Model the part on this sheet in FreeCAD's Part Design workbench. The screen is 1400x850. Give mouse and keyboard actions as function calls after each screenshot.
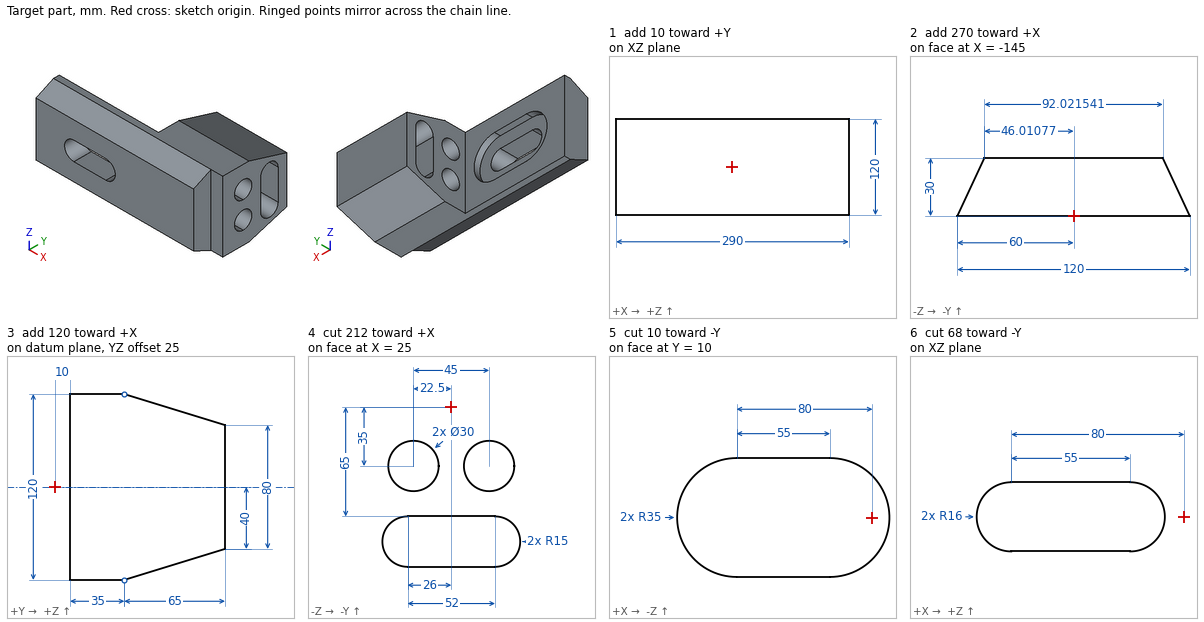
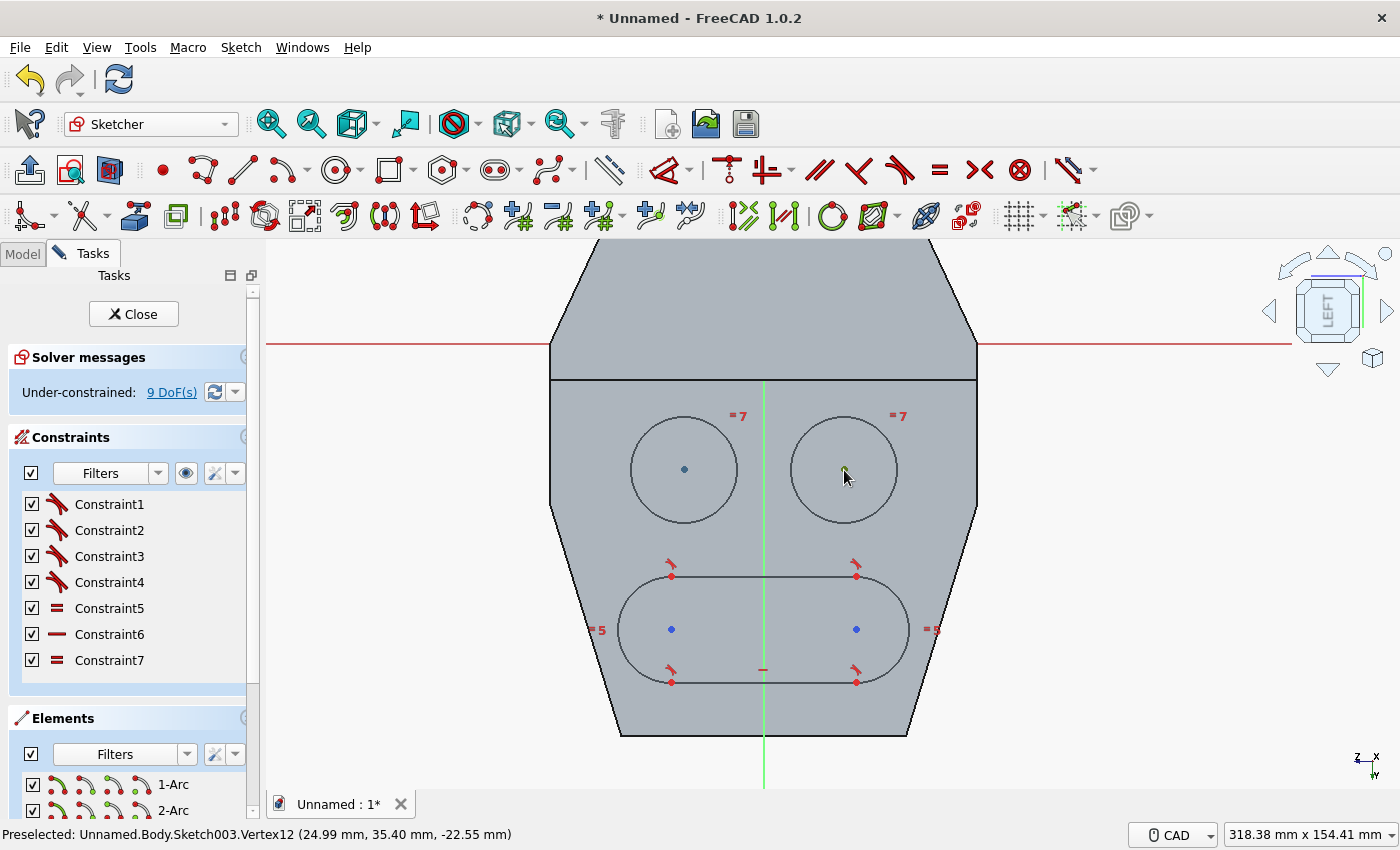
key(h)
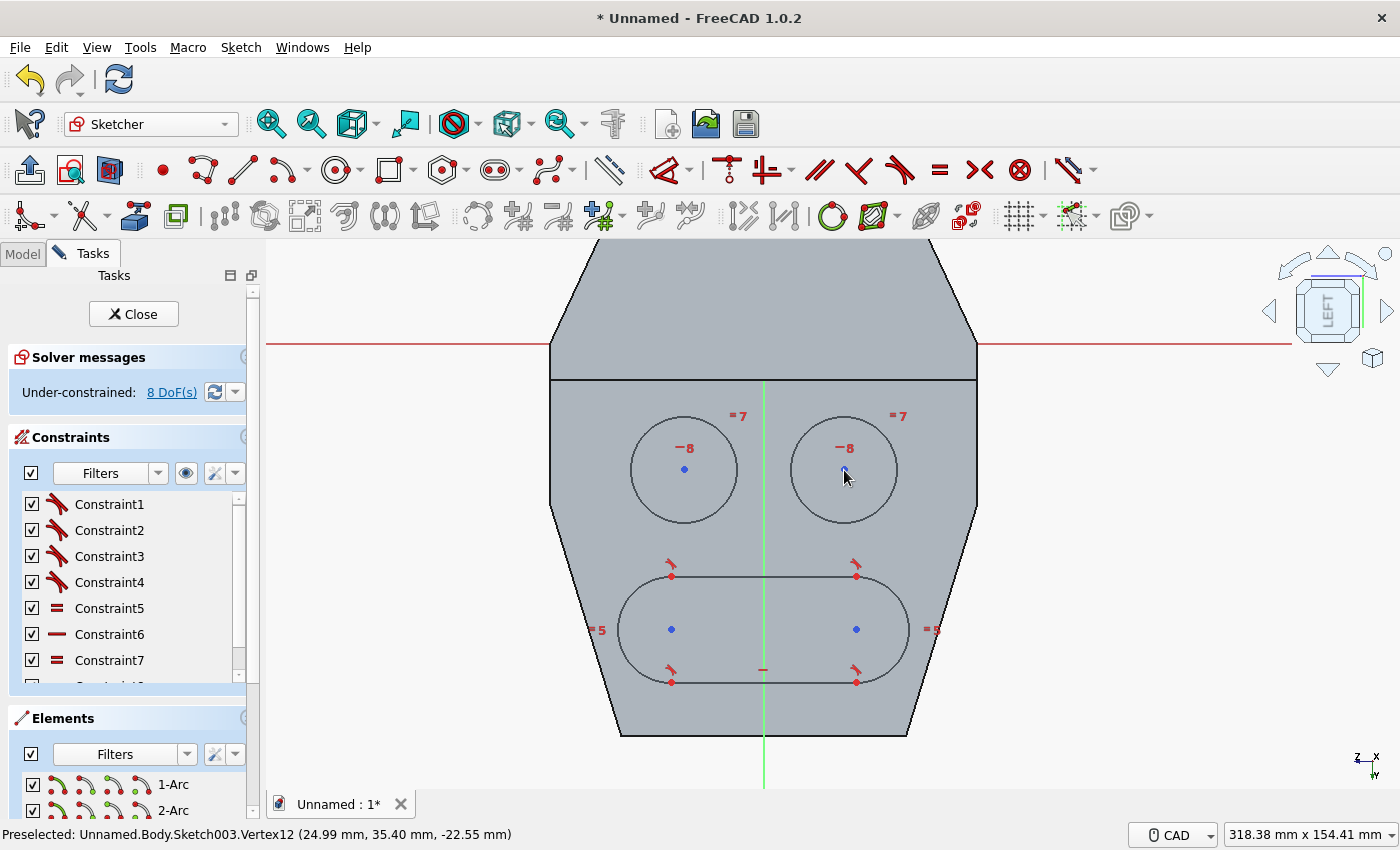
key(d)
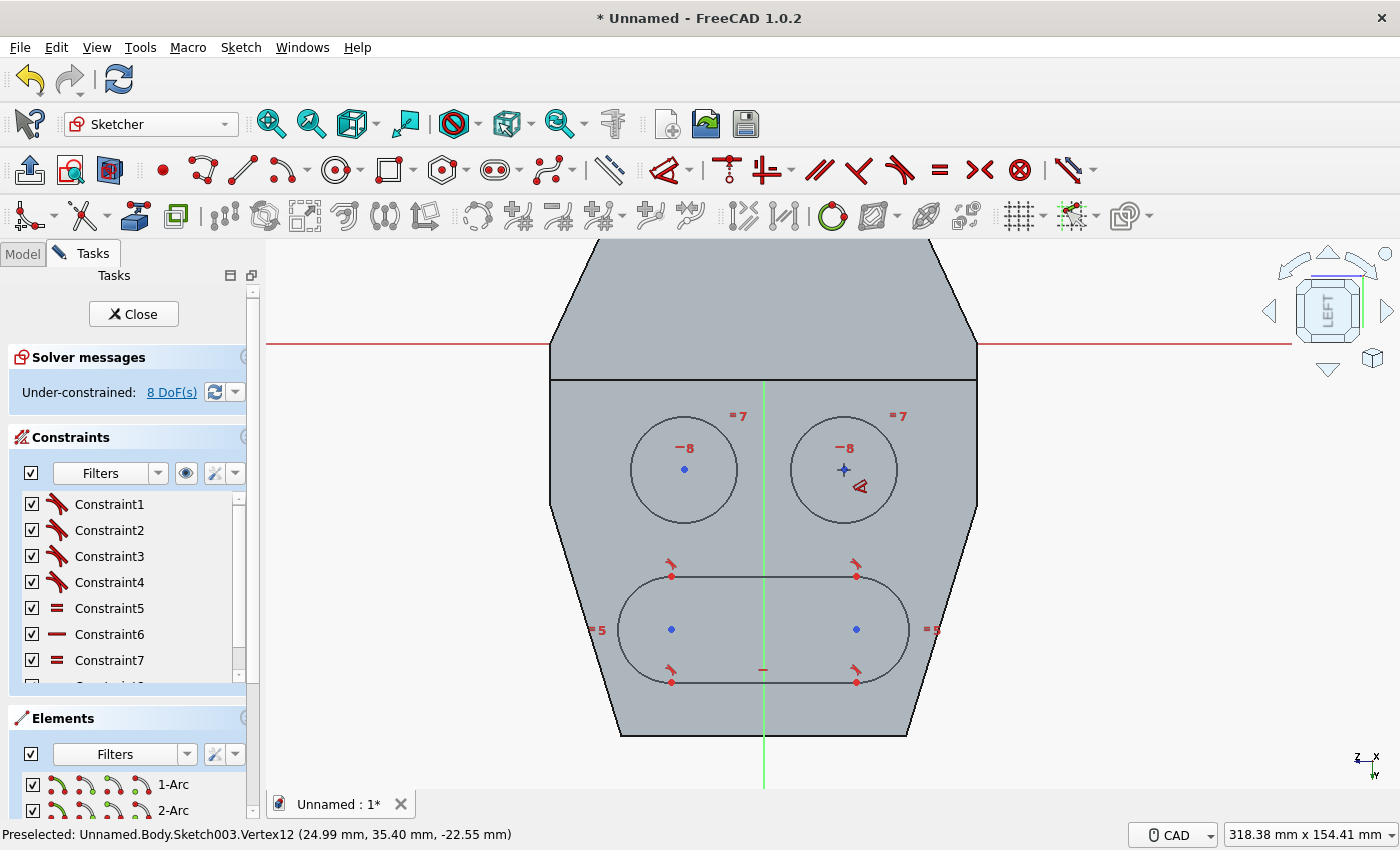
click(628, 599)
click(602, 580)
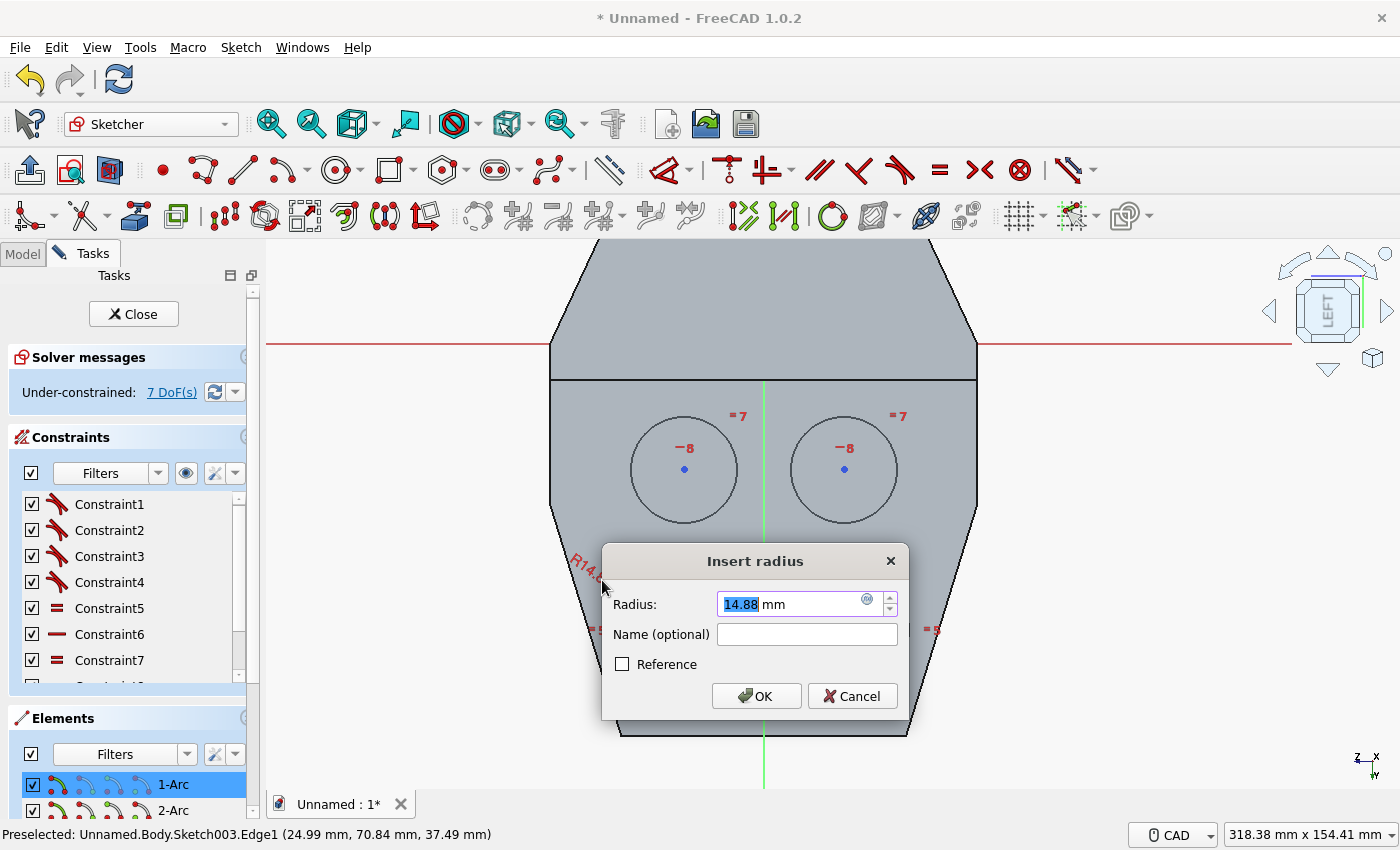
text(15)
key(Return)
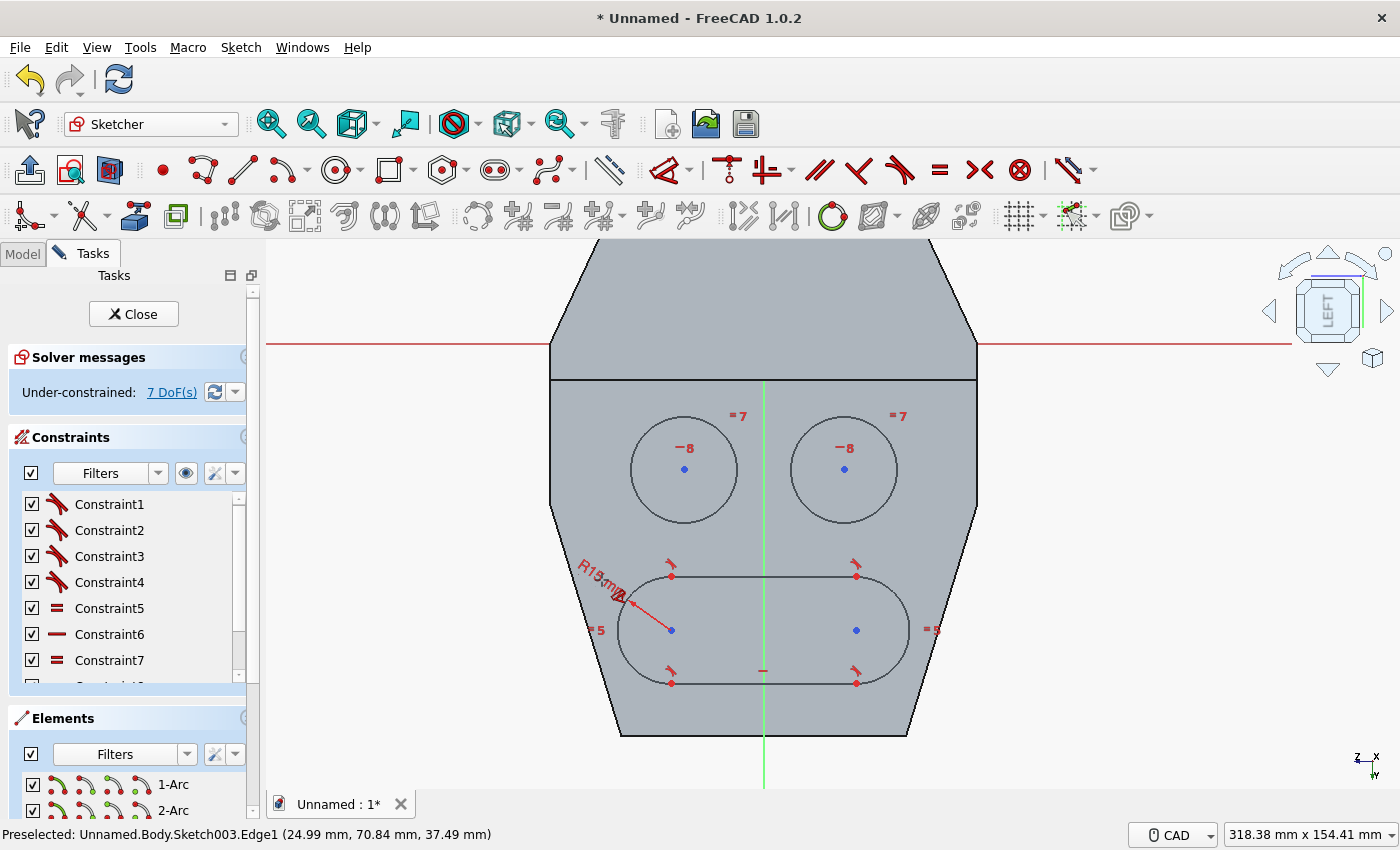
click(721, 432)
click(743, 409)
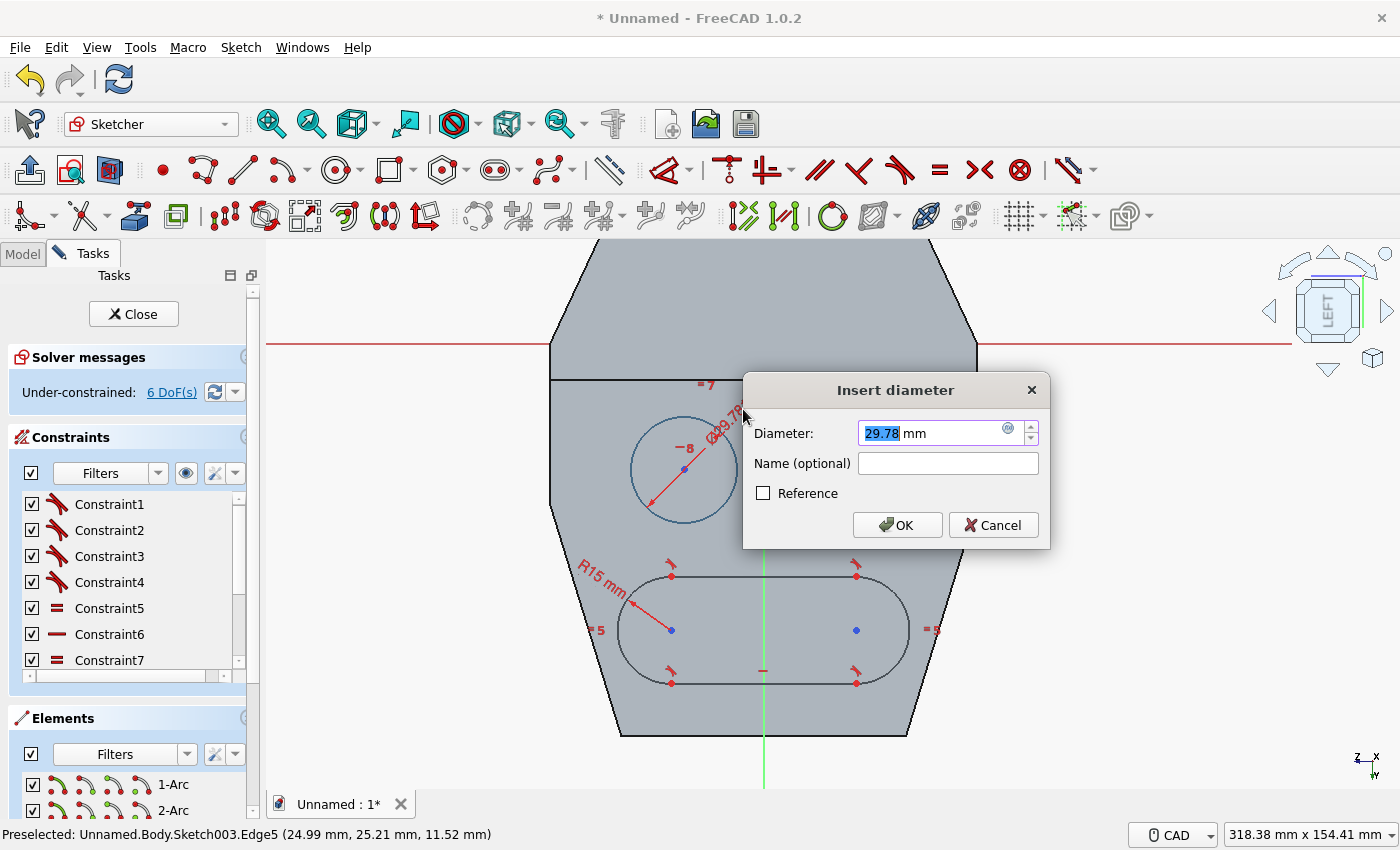
text(30)
key(Return)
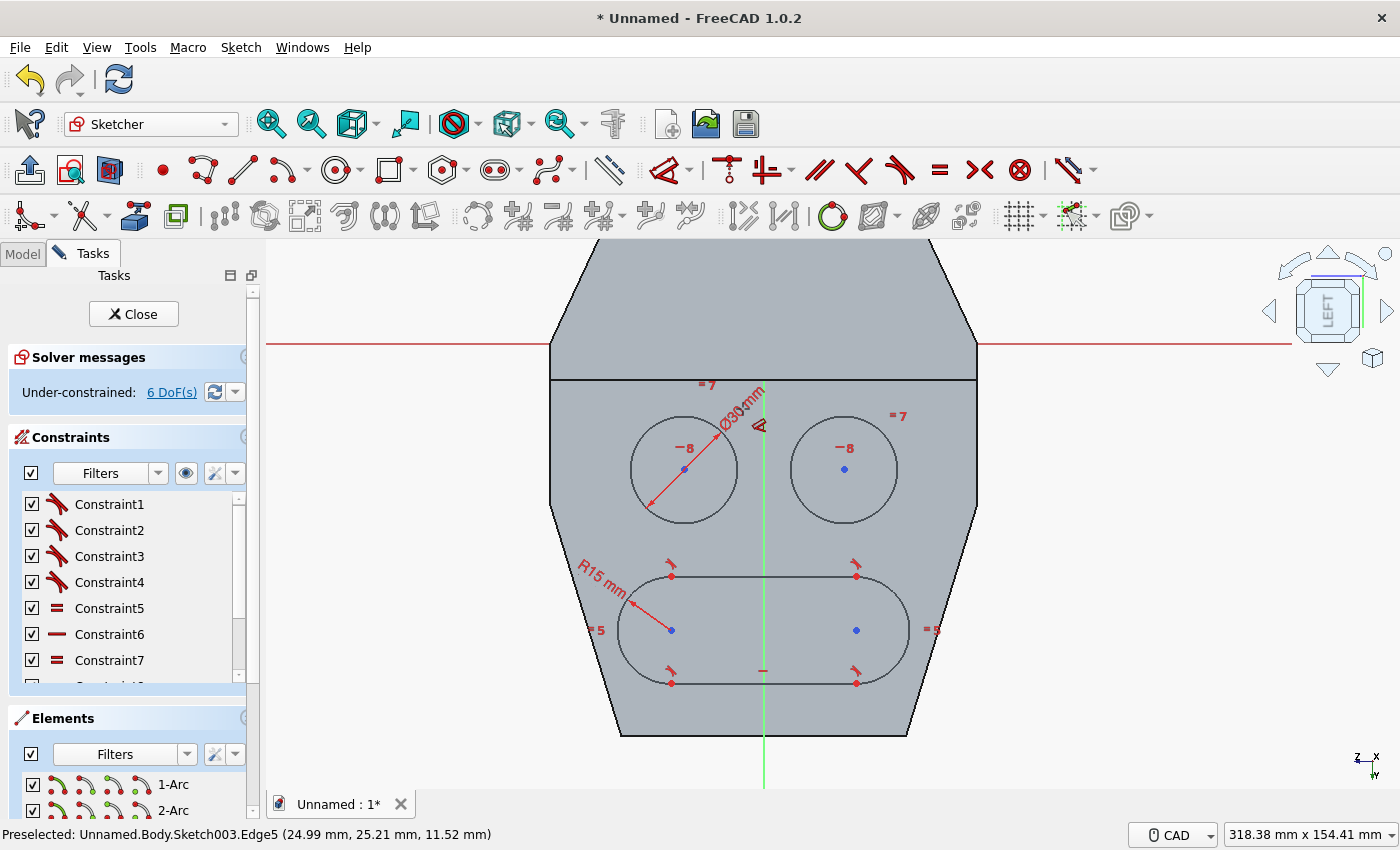
click(727, 577)
click(721, 611)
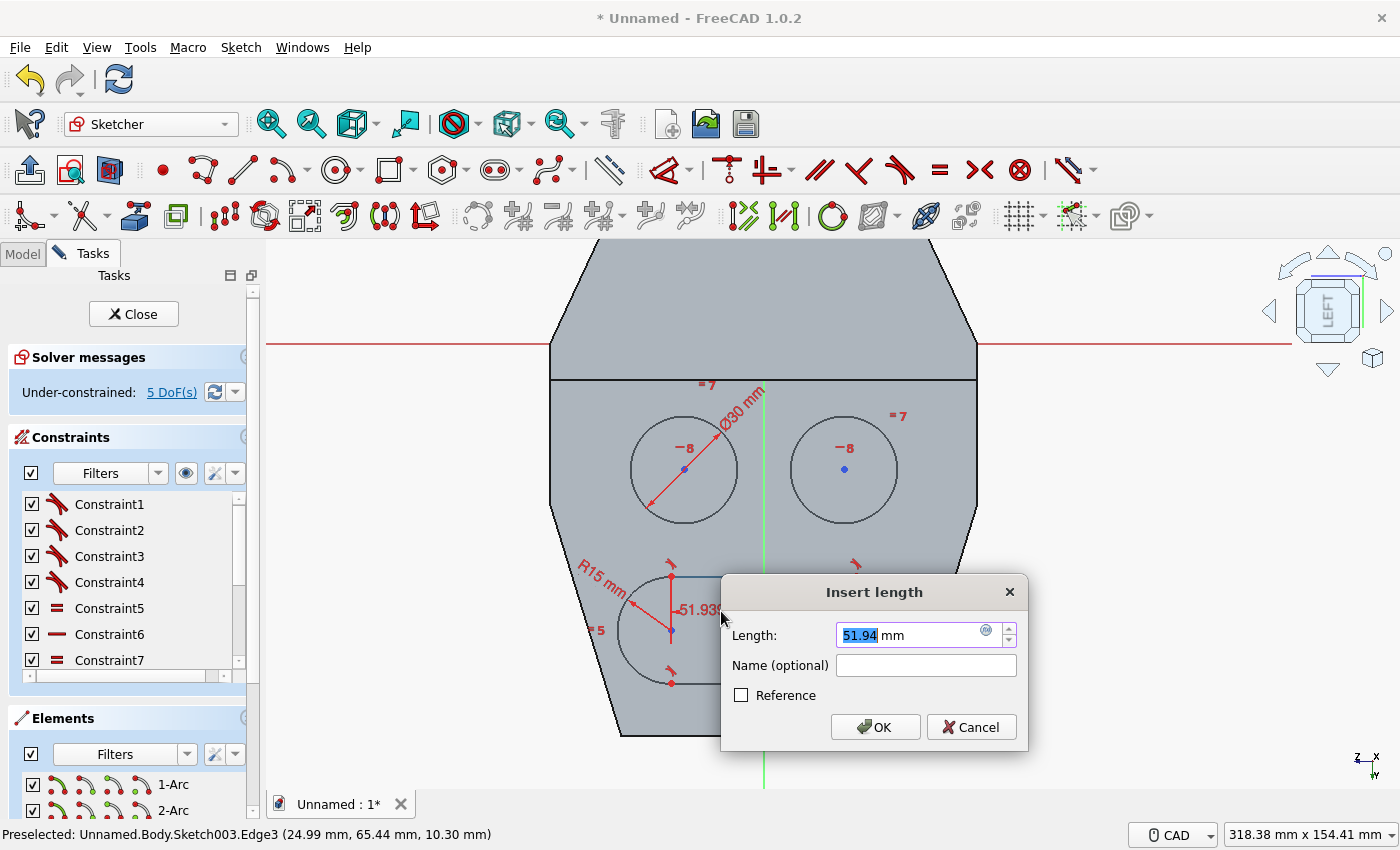
text(52)
key(Return)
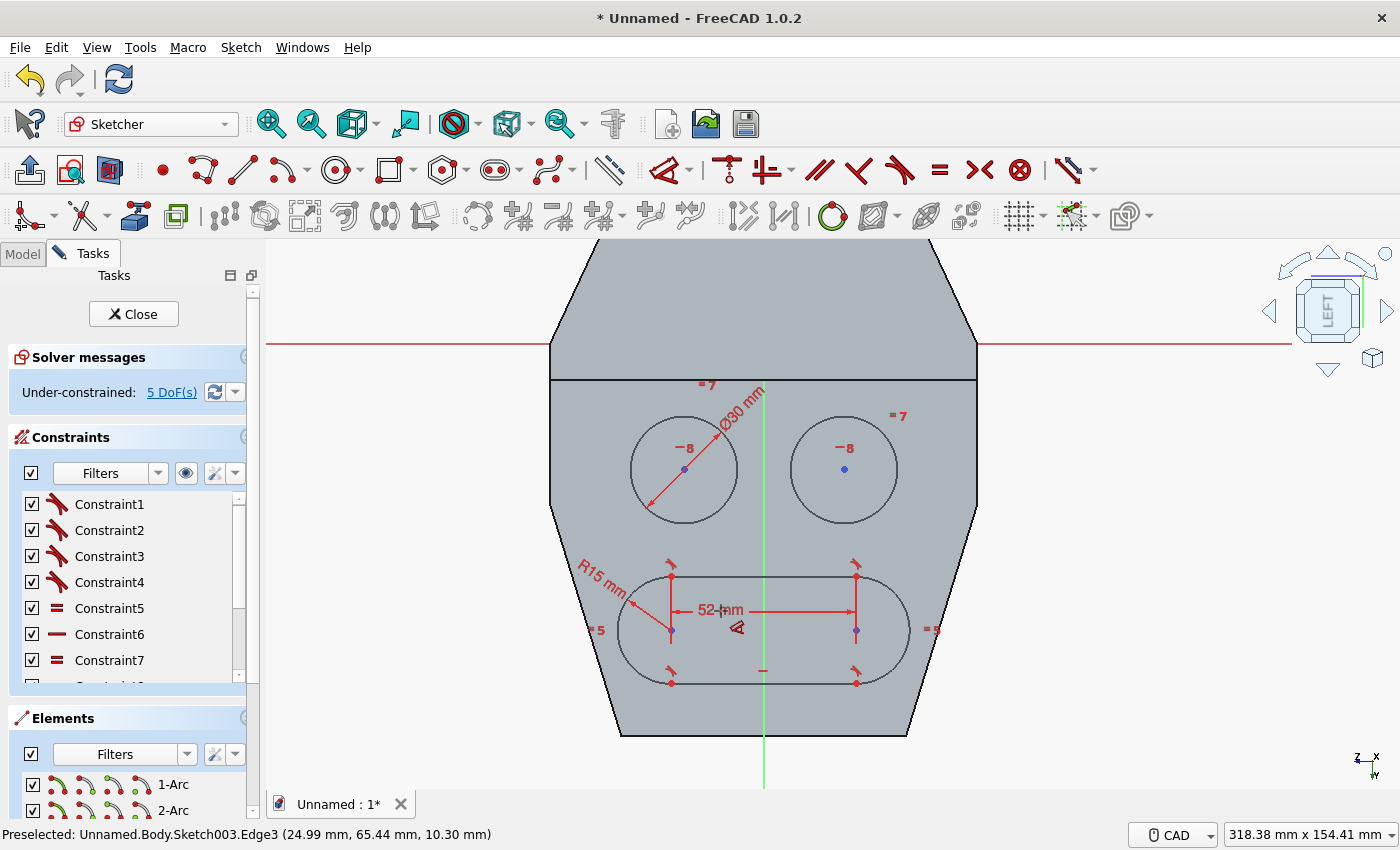
click(684, 470)
click(650, 407)